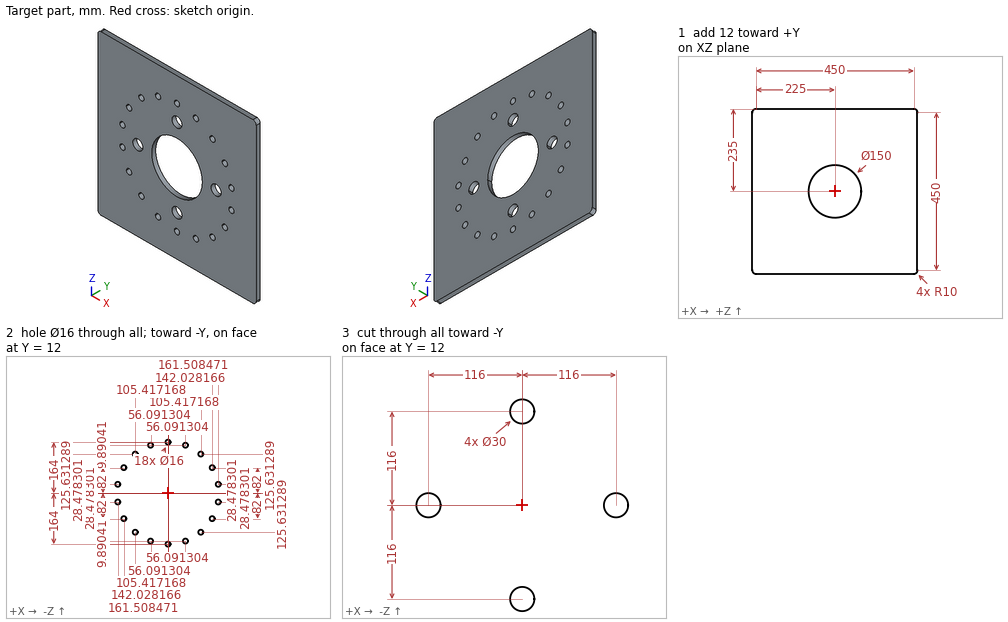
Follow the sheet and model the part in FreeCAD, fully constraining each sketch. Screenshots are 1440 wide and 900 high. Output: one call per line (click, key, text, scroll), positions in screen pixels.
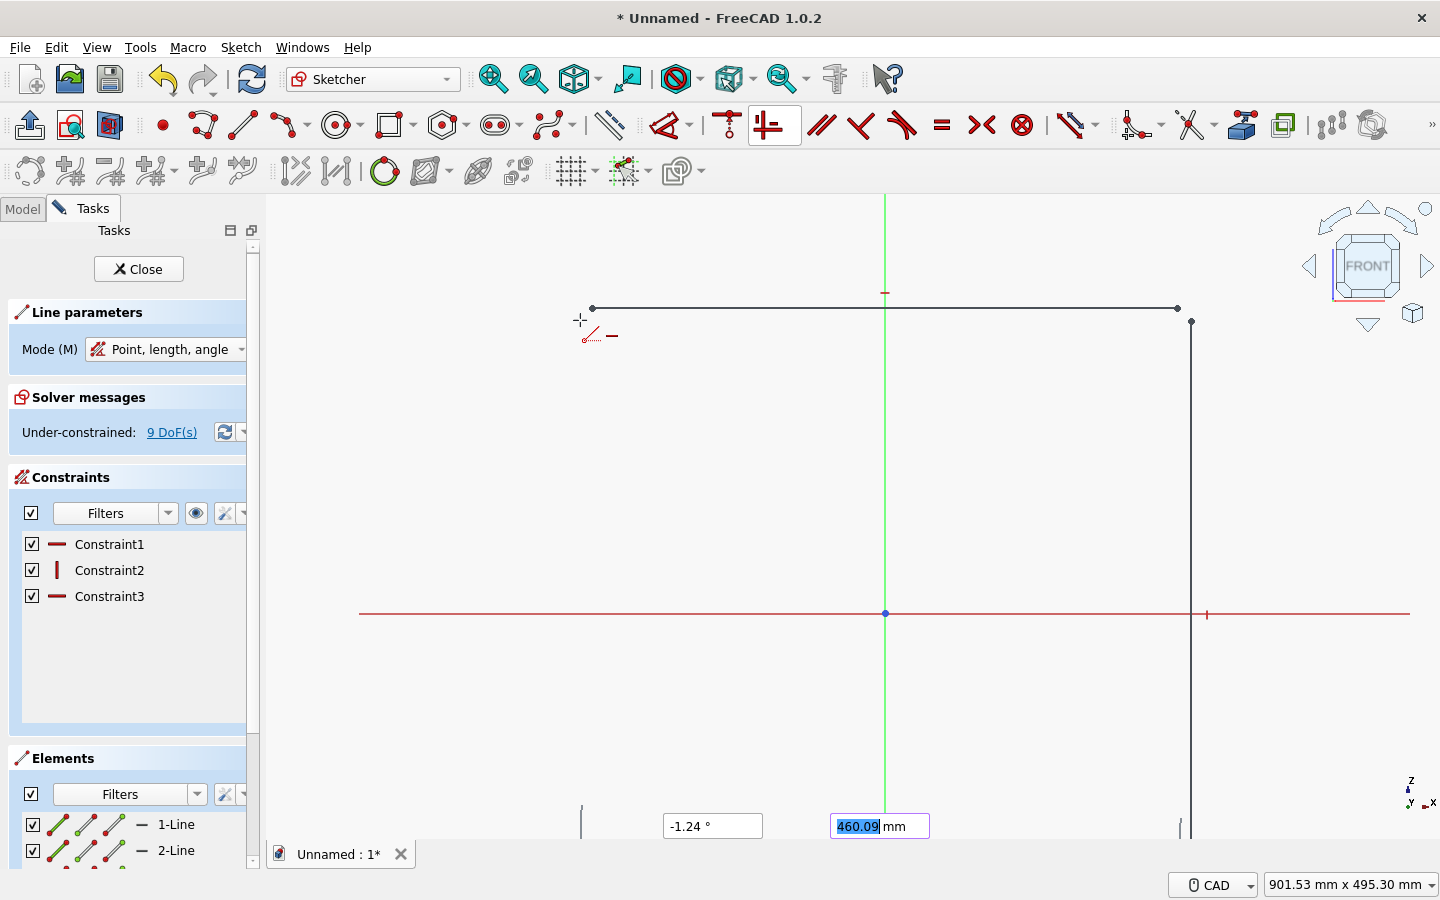
click(579, 321)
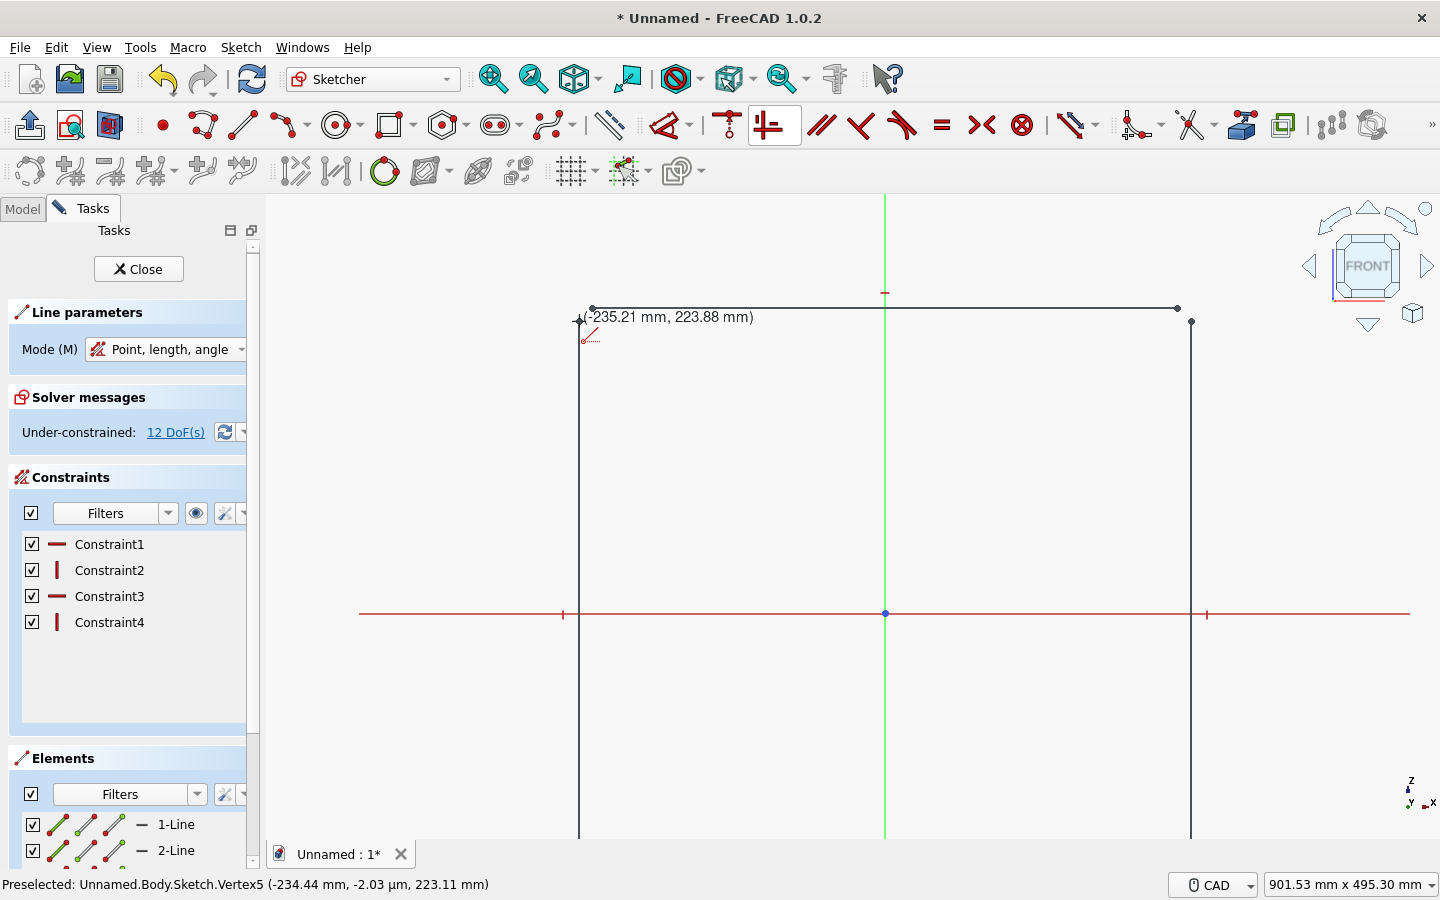
click(284, 126)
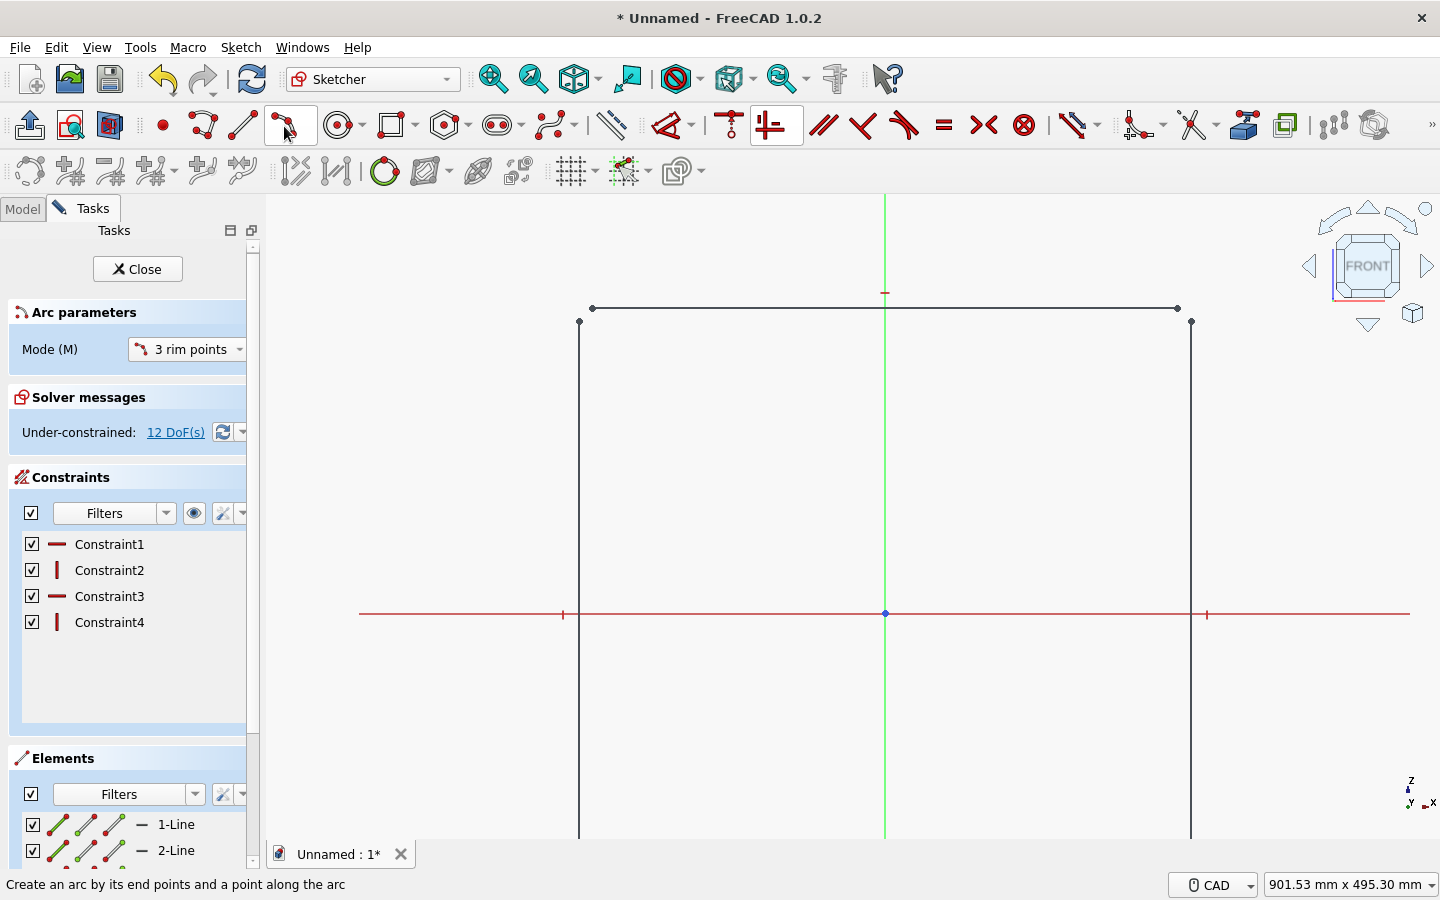
click(1178, 308)
click(1191, 321)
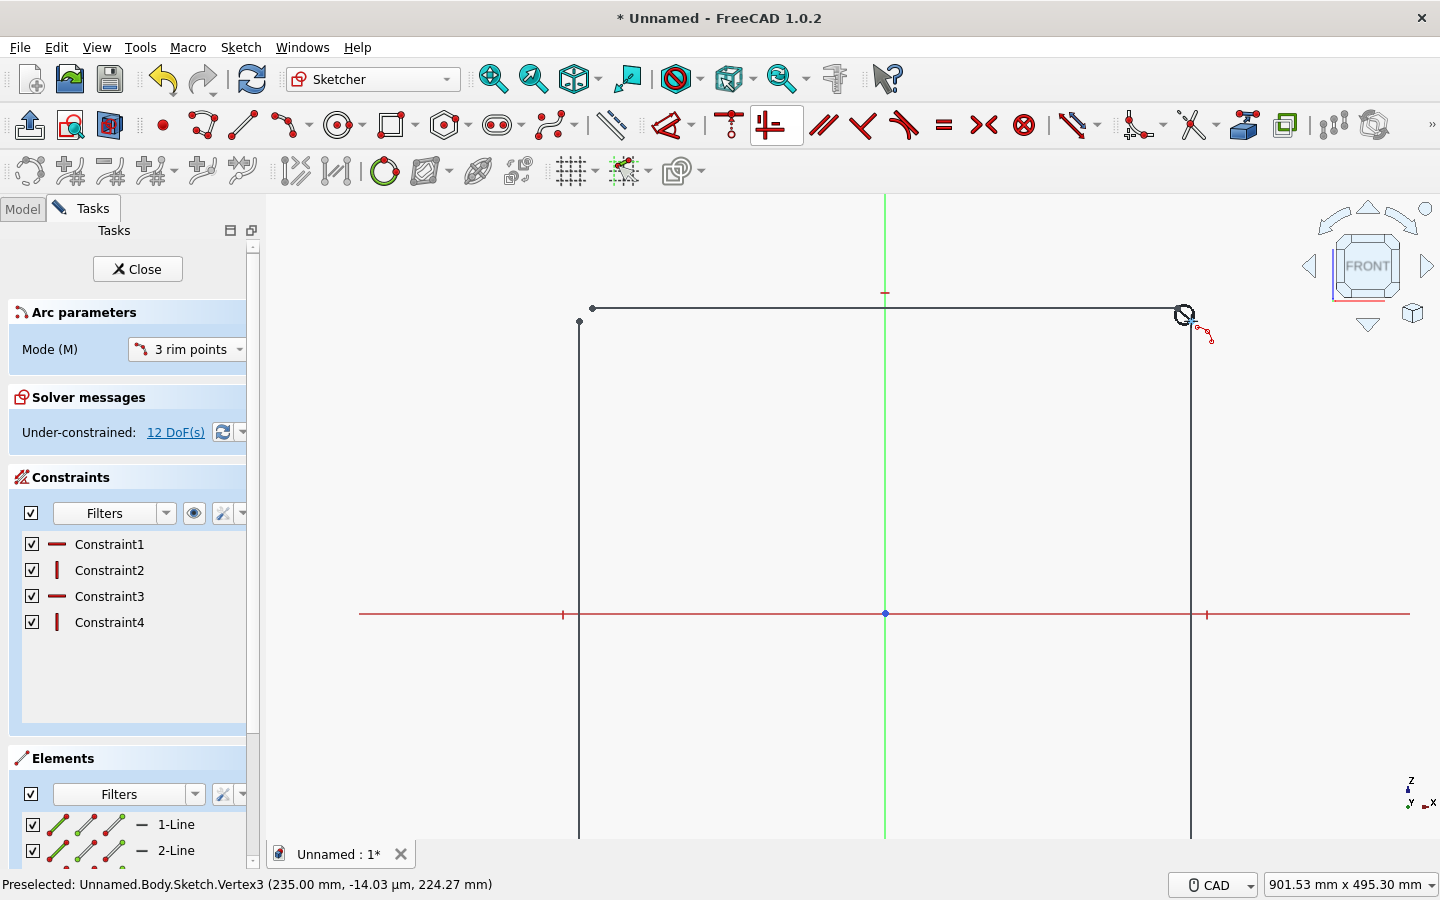
scroll(1188, 311, up, 8)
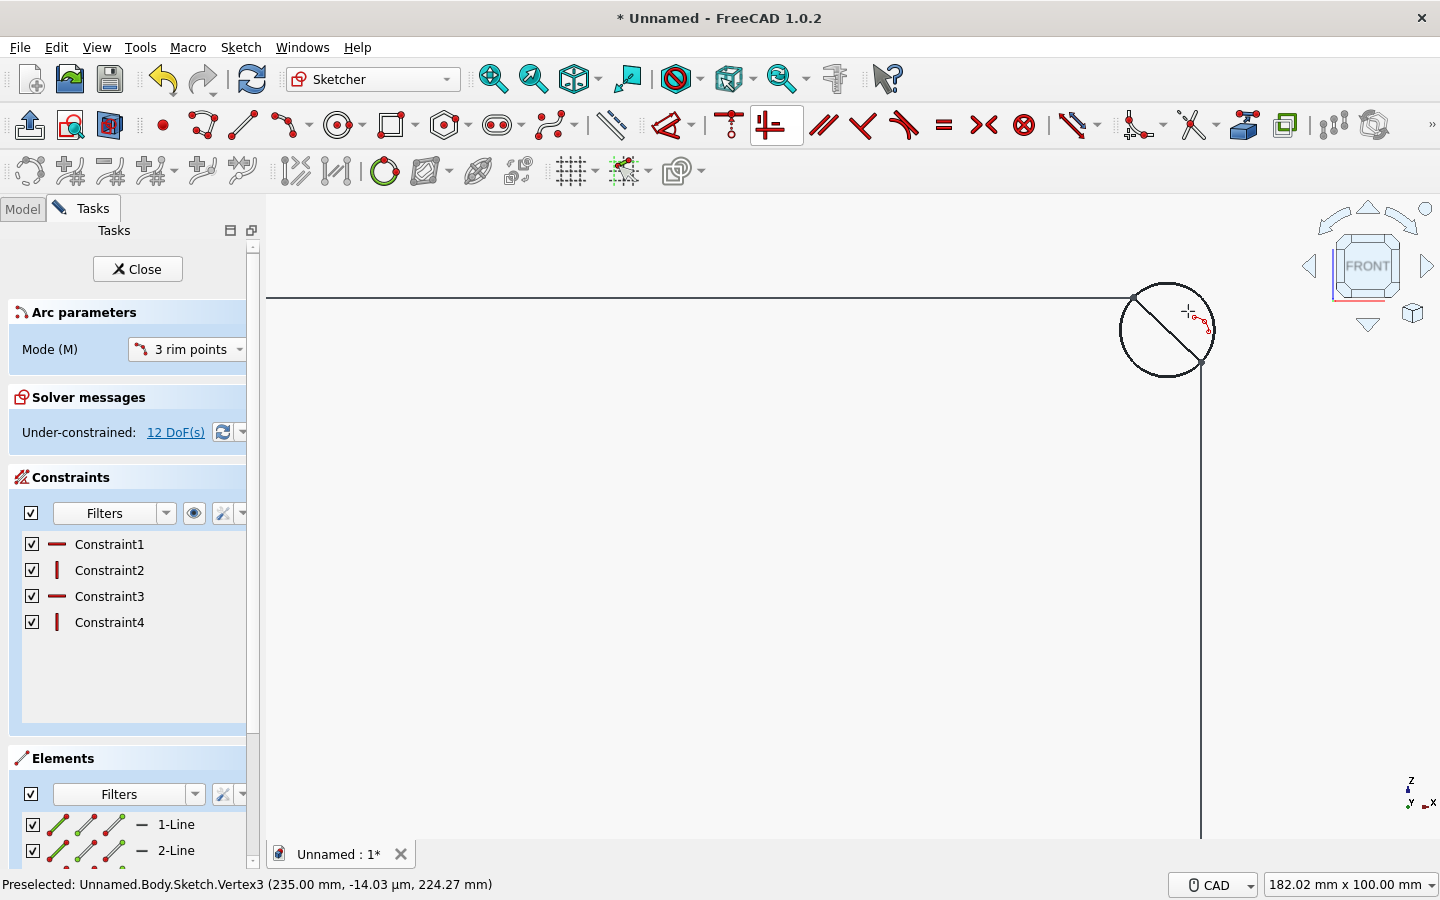
click(1182, 312)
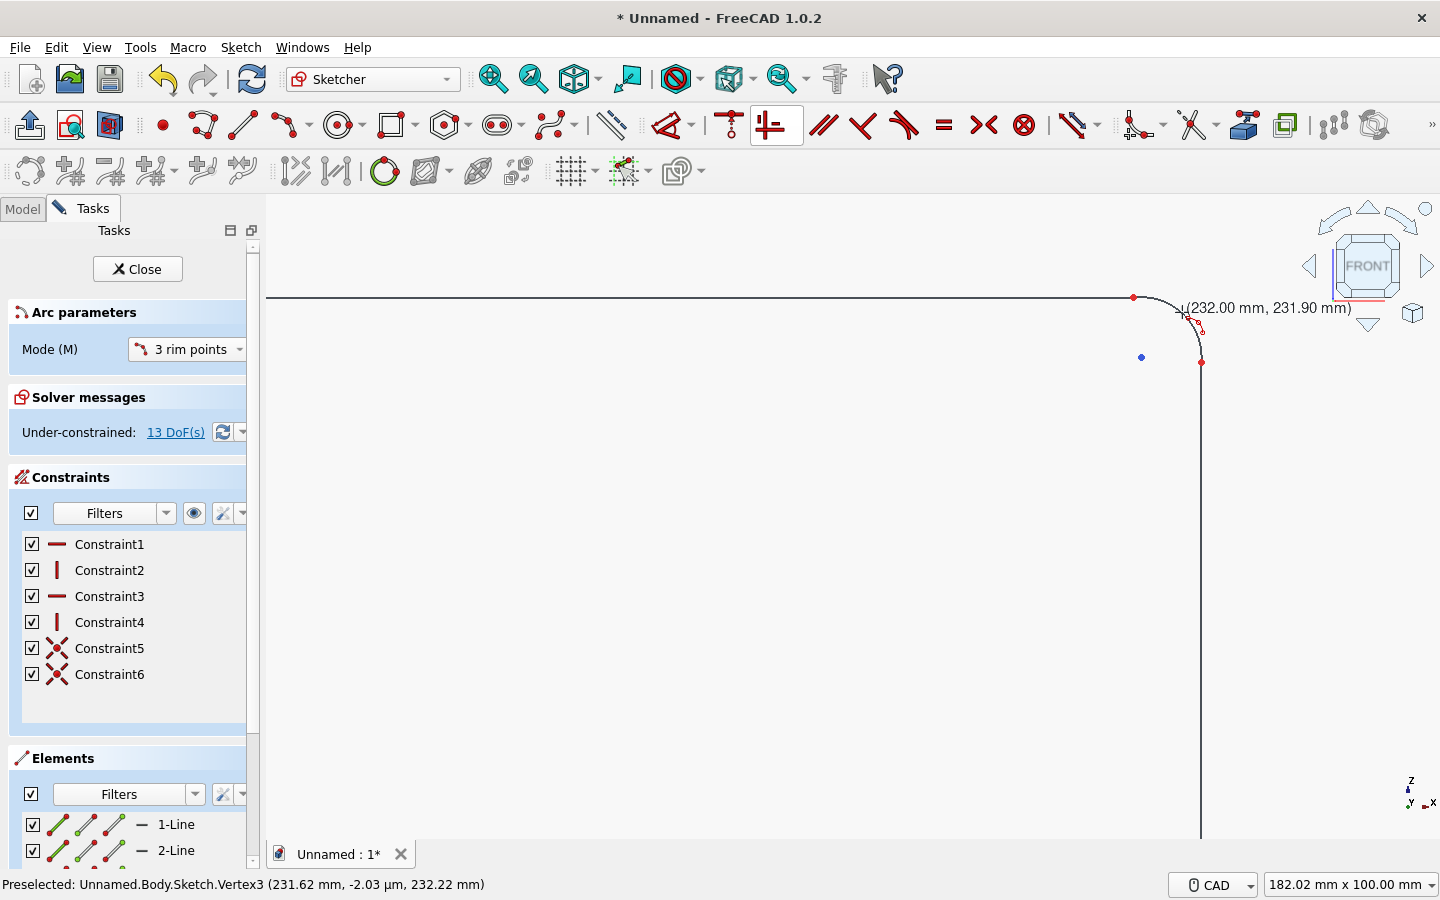
scroll(956, 314, down, 10)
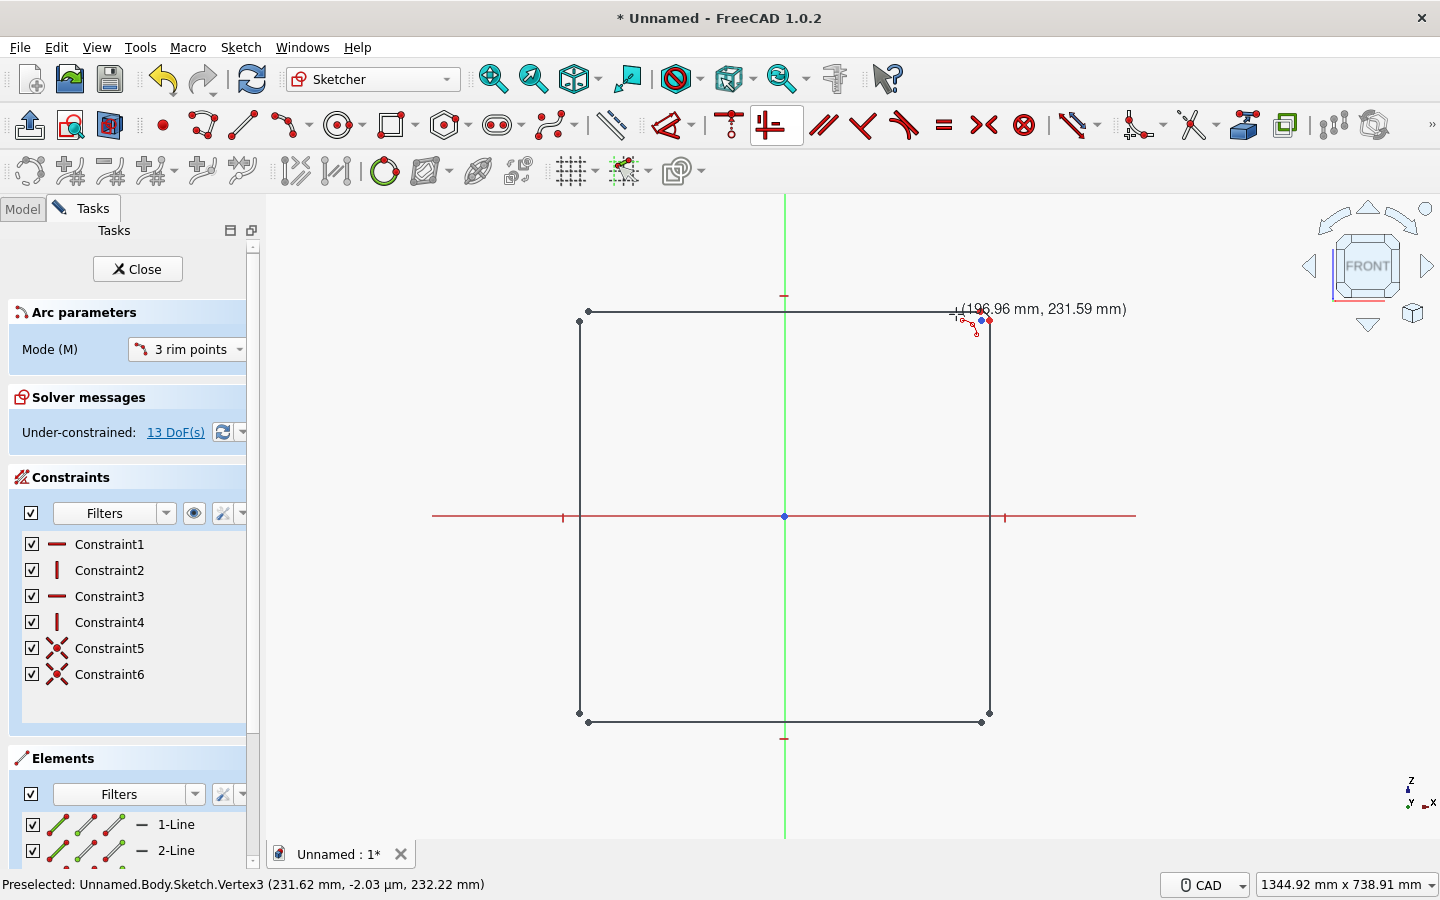
scroll(990, 713, up, 2)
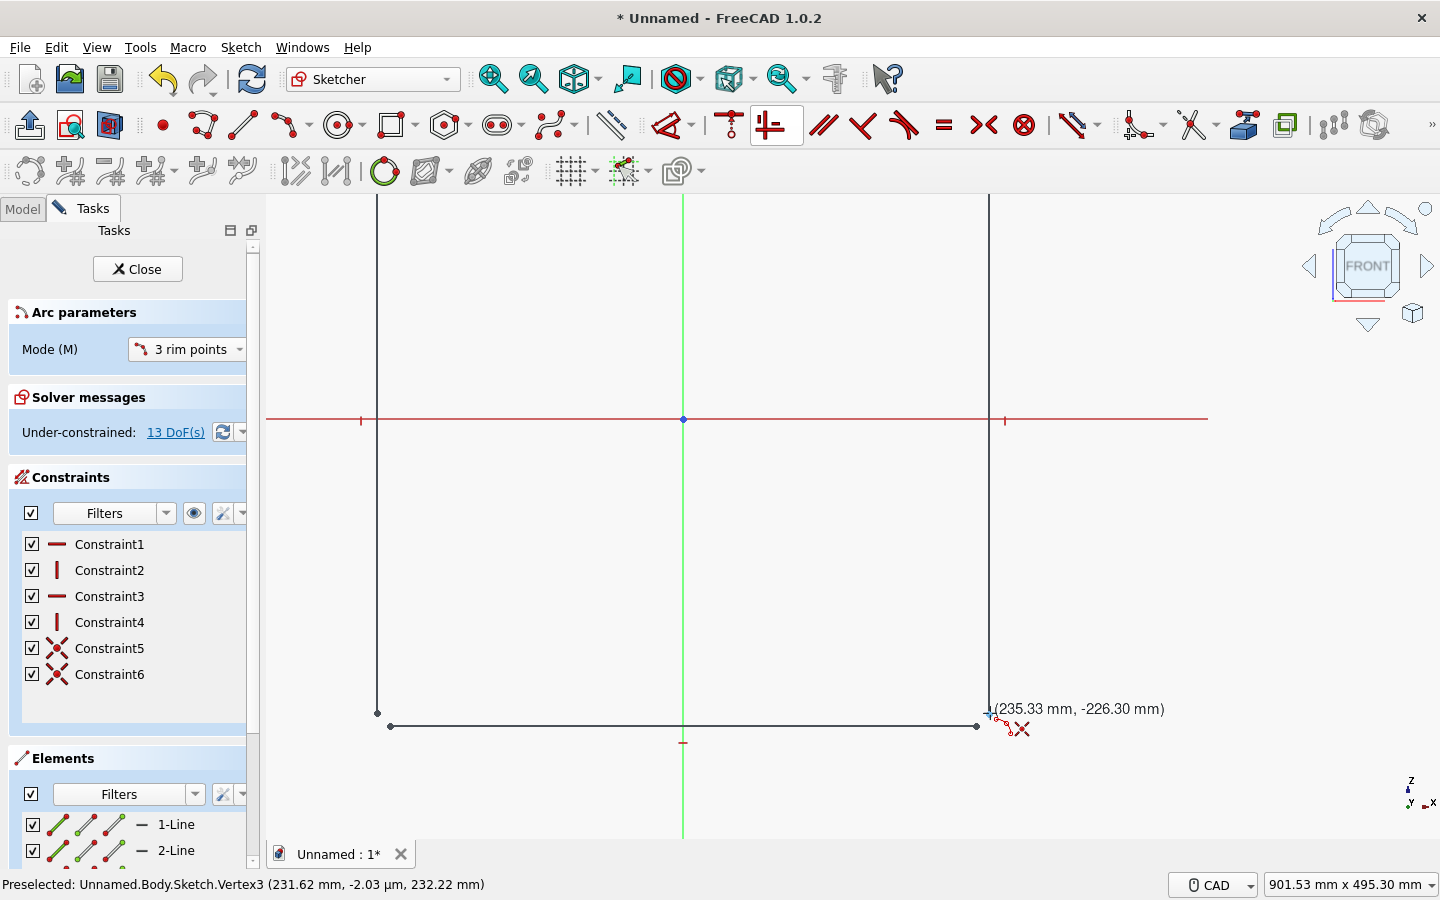
click(989, 714)
click(976, 726)